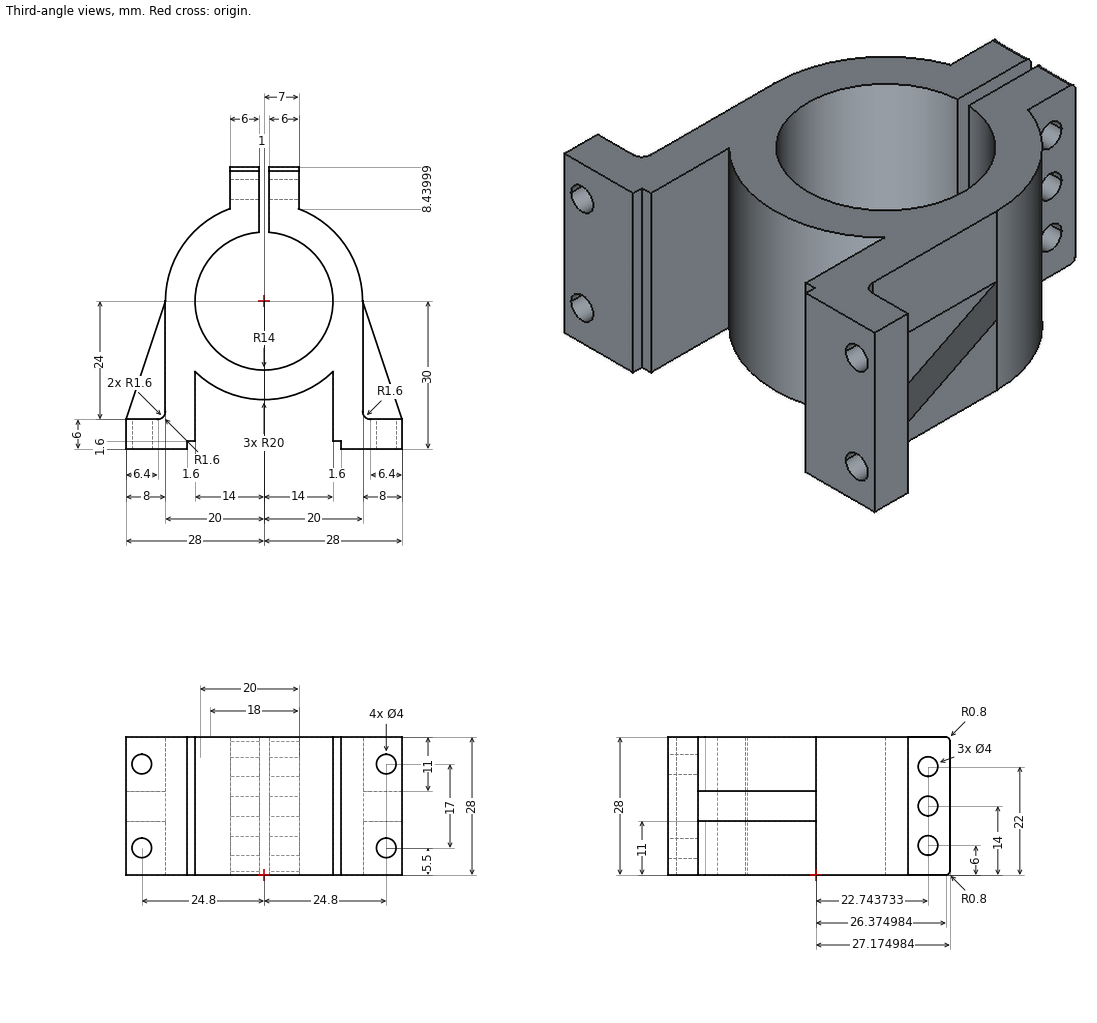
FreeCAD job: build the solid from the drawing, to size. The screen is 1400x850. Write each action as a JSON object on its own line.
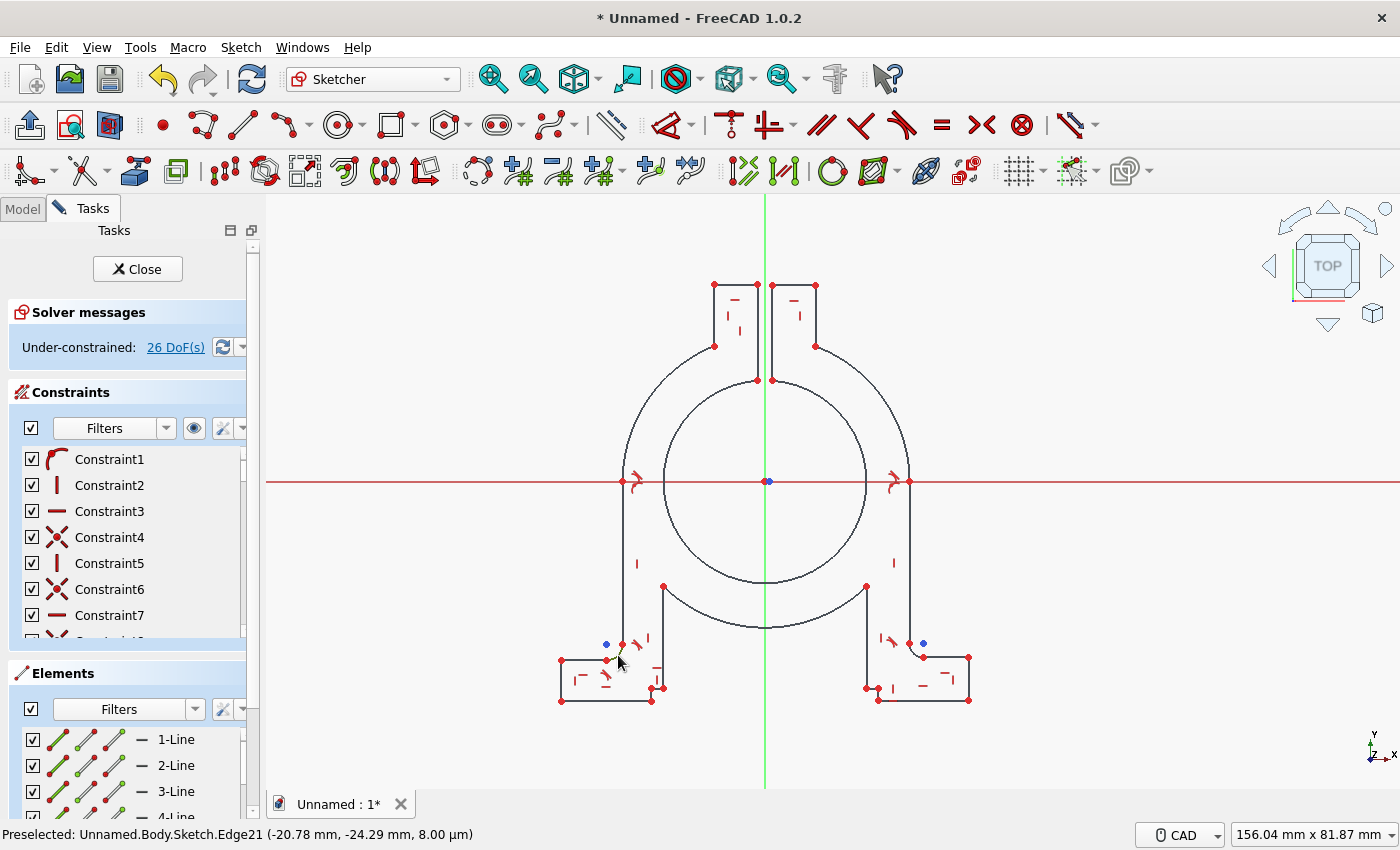
{"action": "scroll", "coordinate": [914, 654], "scroll_direction": "up", "scroll_amount": 2}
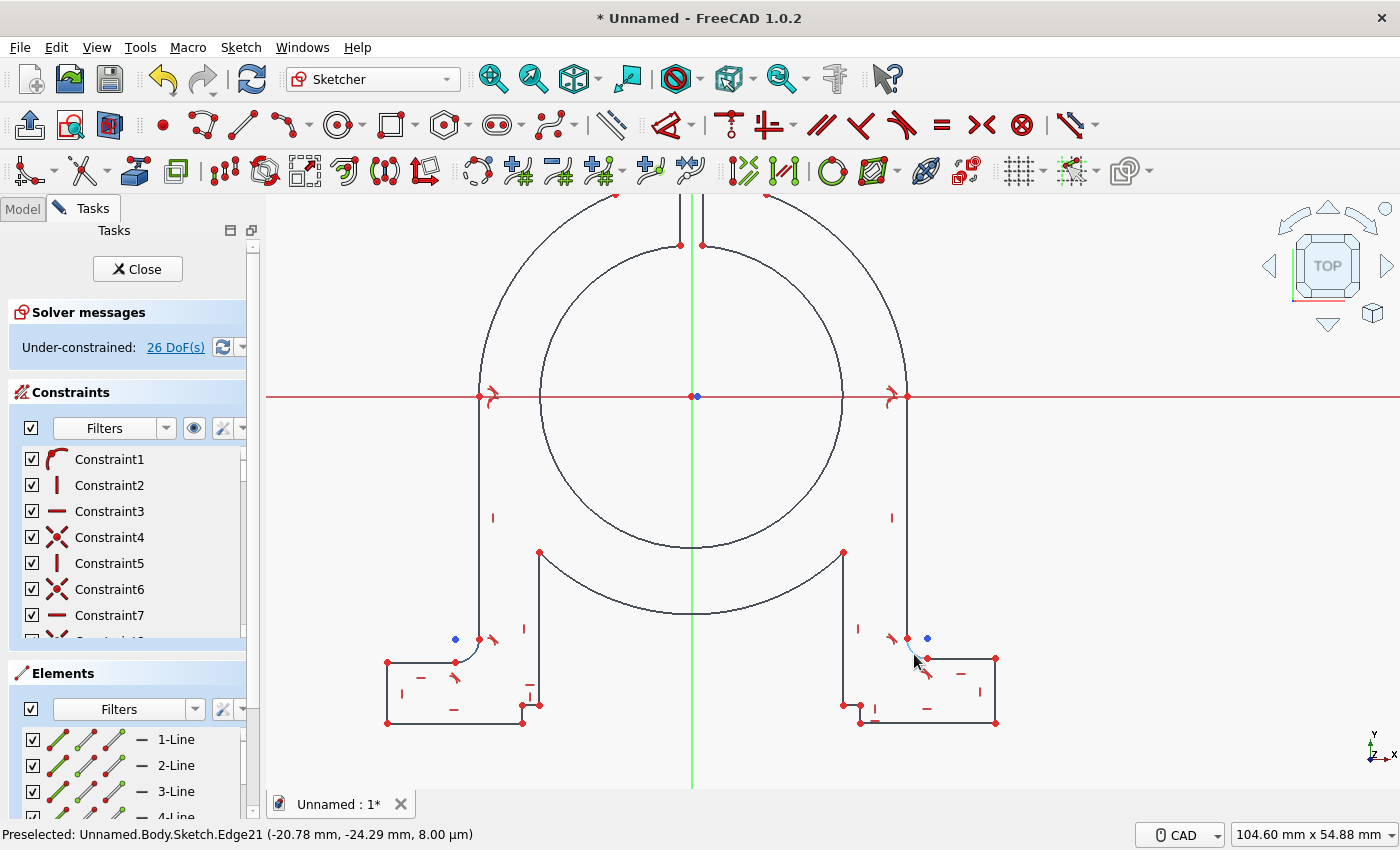
{"action": "left_click", "coordinate": [913, 653]}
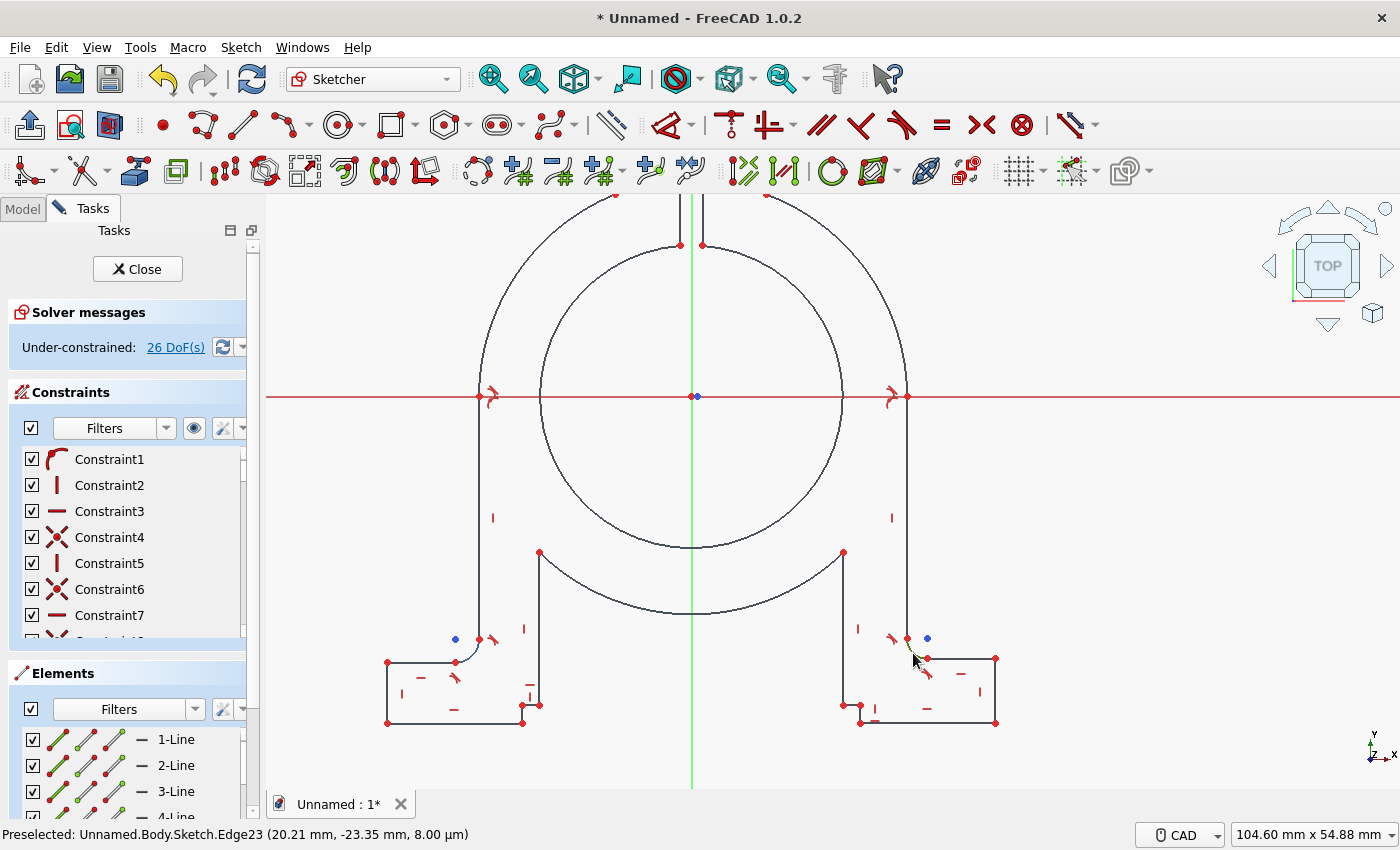
{"action": "left_click", "coordinate": [942, 126]}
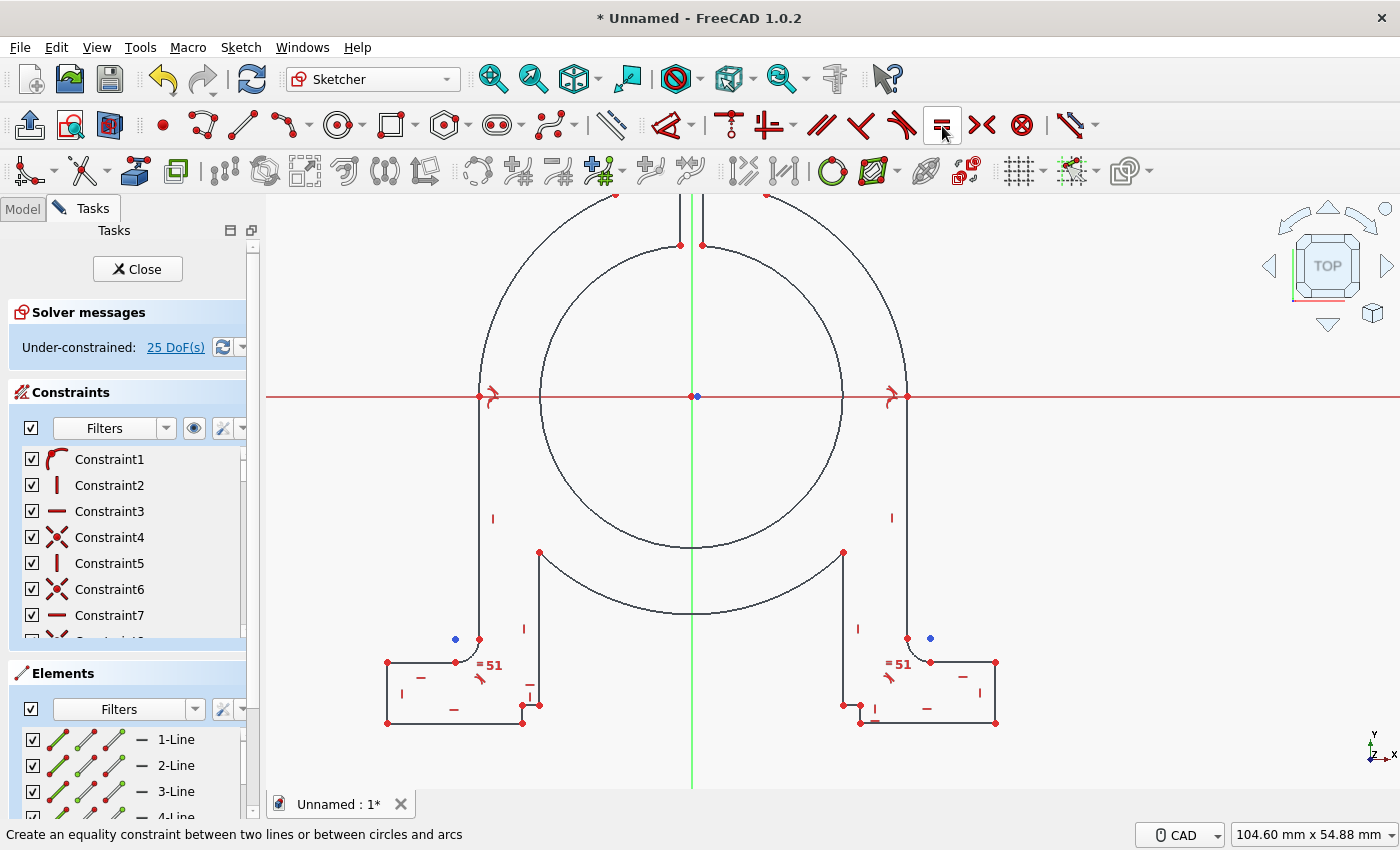
{"action": "left_click", "coordinate": [625, 604]}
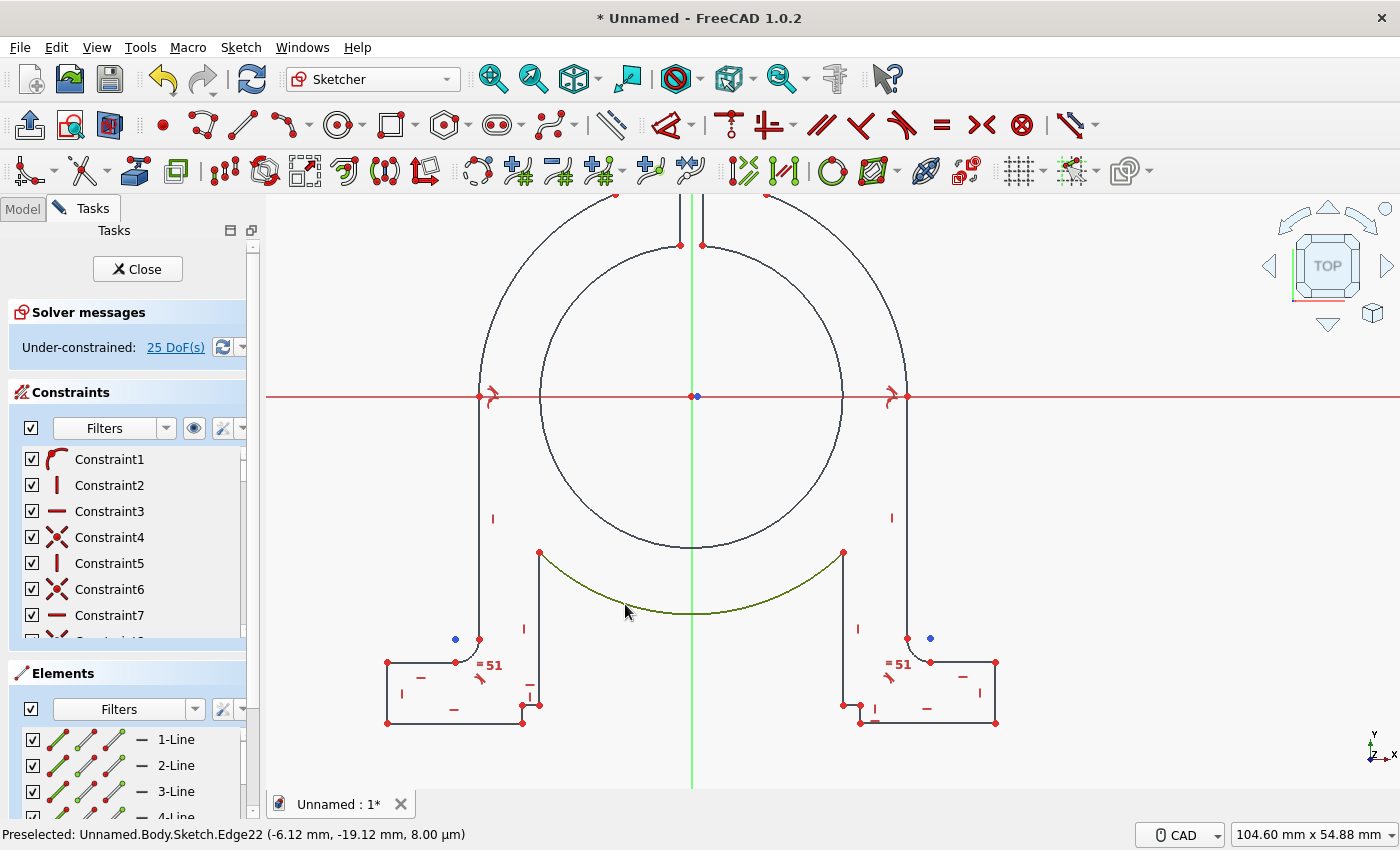
{"action": "left_click", "coordinate": [893, 320]}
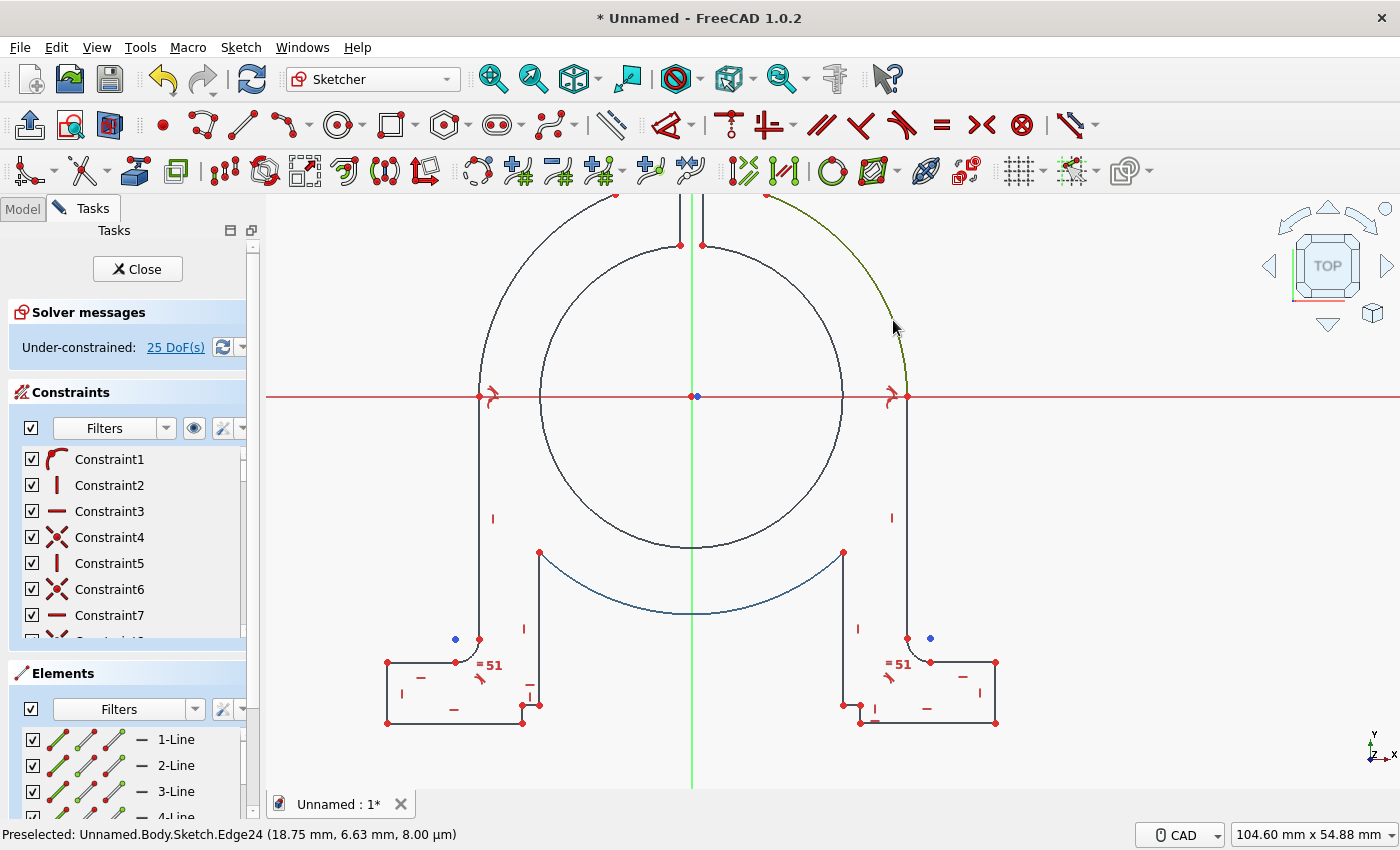
{"action": "left_click", "coordinate": [550, 236]}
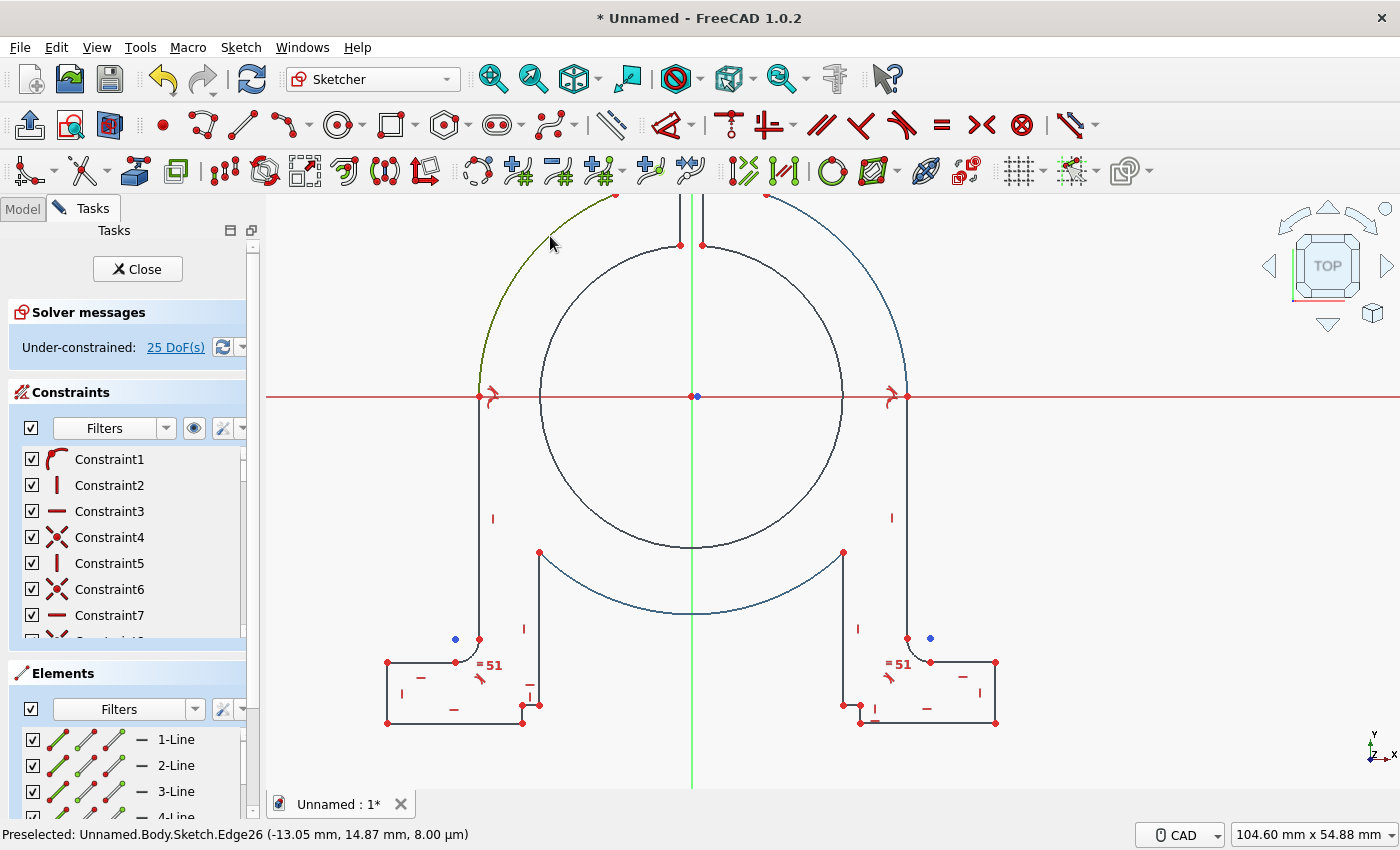
{"action": "left_click", "coordinate": [942, 126]}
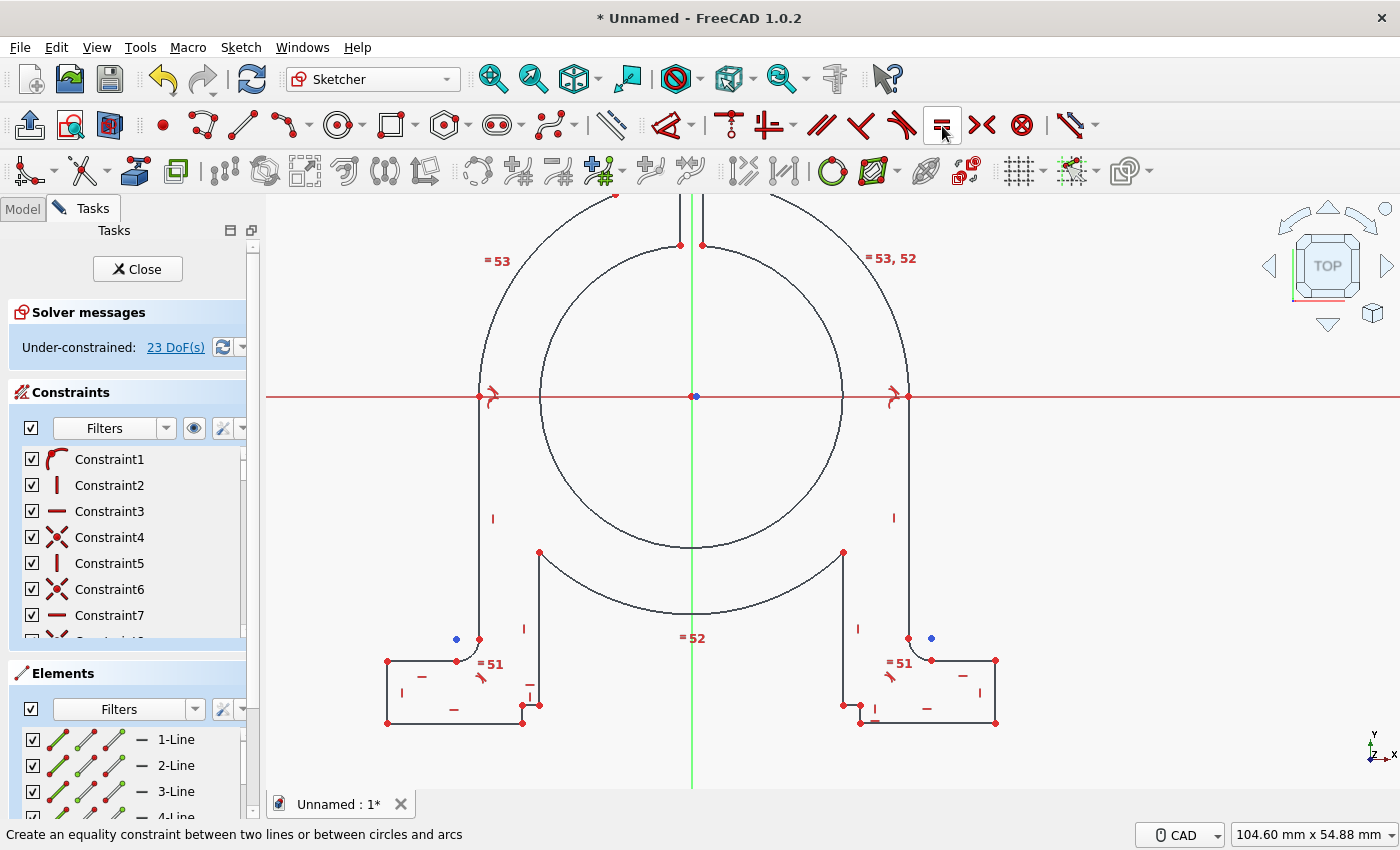
{"action": "left_click", "coordinate": [691, 397]}